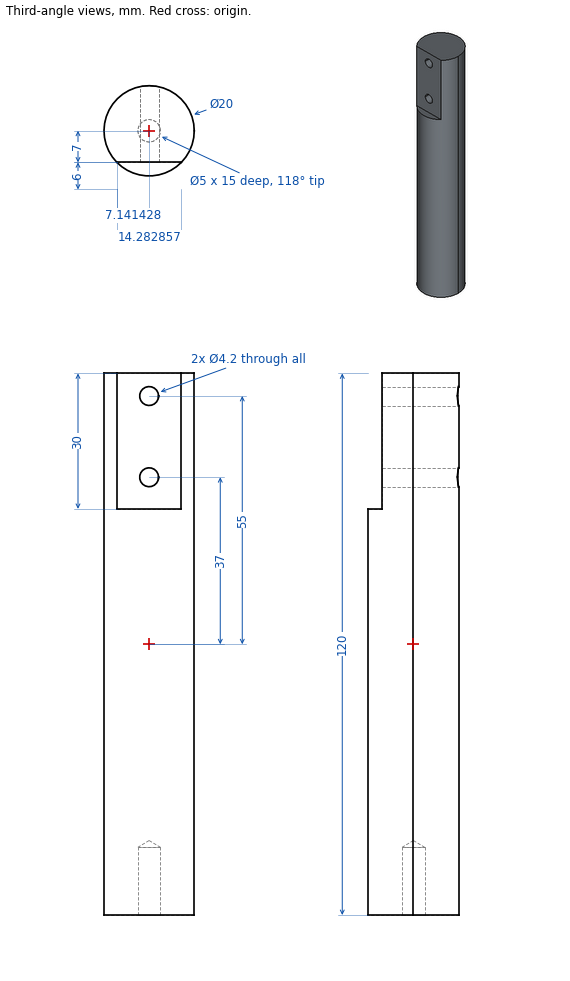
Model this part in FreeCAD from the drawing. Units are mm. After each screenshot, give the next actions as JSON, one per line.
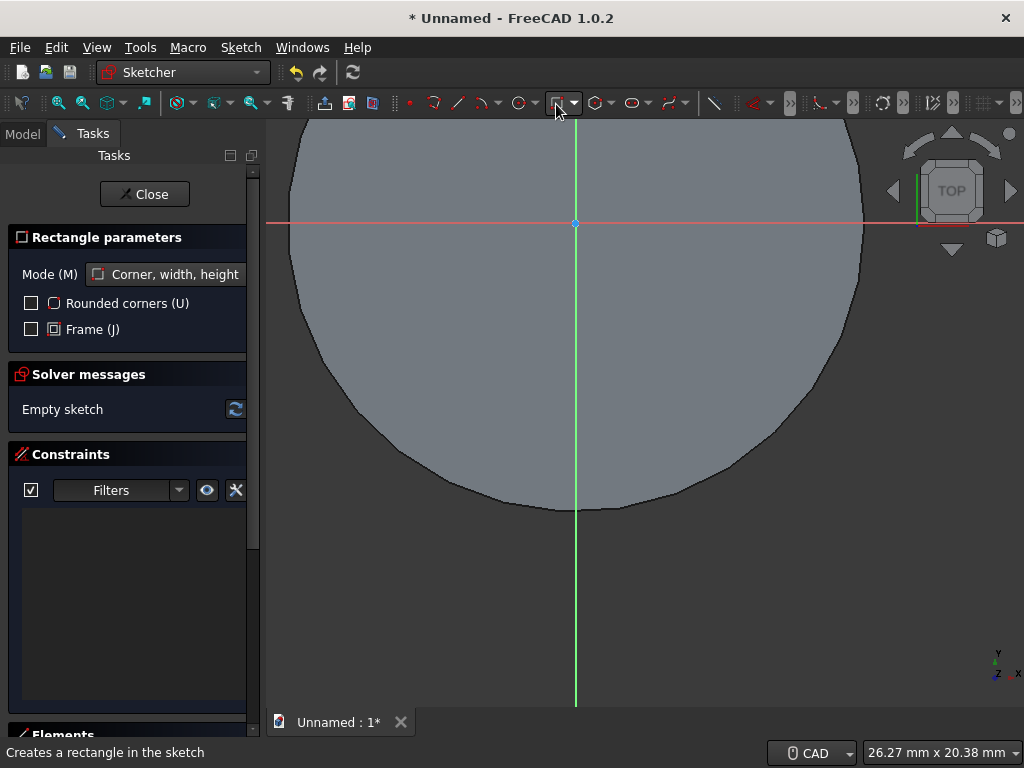
{"action": "left_click", "coordinate": [370, 425]}
{"action": "left_click", "coordinate": [782, 598]}
{"action": "key", "text": "Escape"}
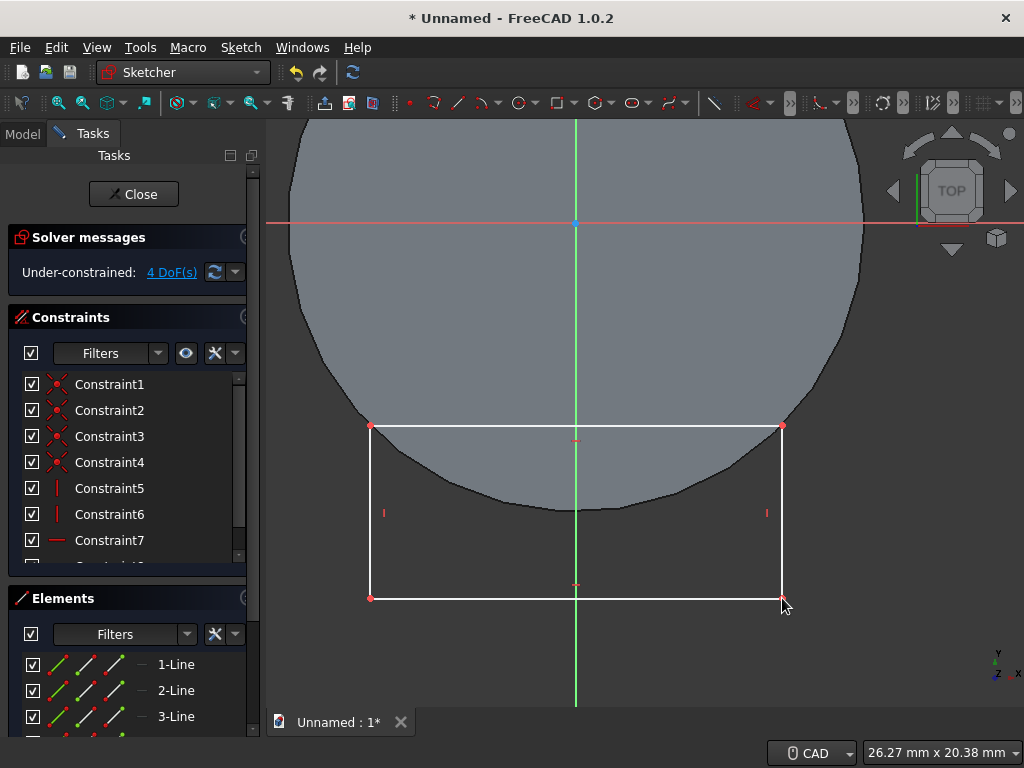
{"action": "left_click", "coordinate": [754, 104]}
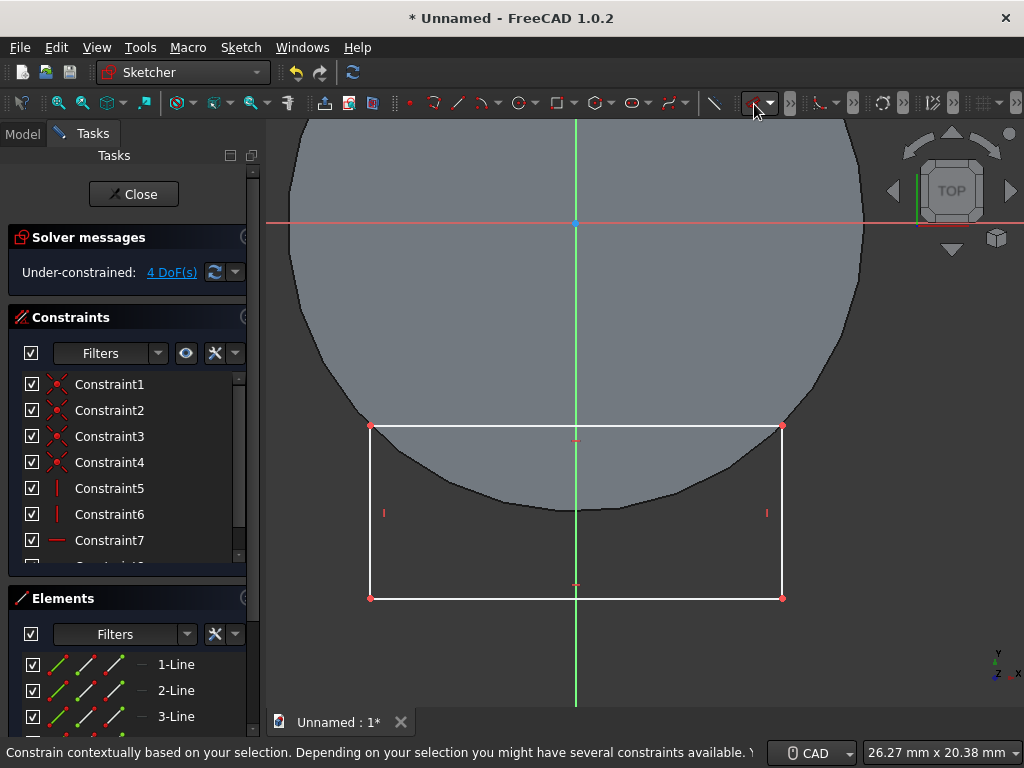
{"action": "left_click", "coordinate": [370, 478]}
{"action": "left_click", "coordinate": [336, 513]}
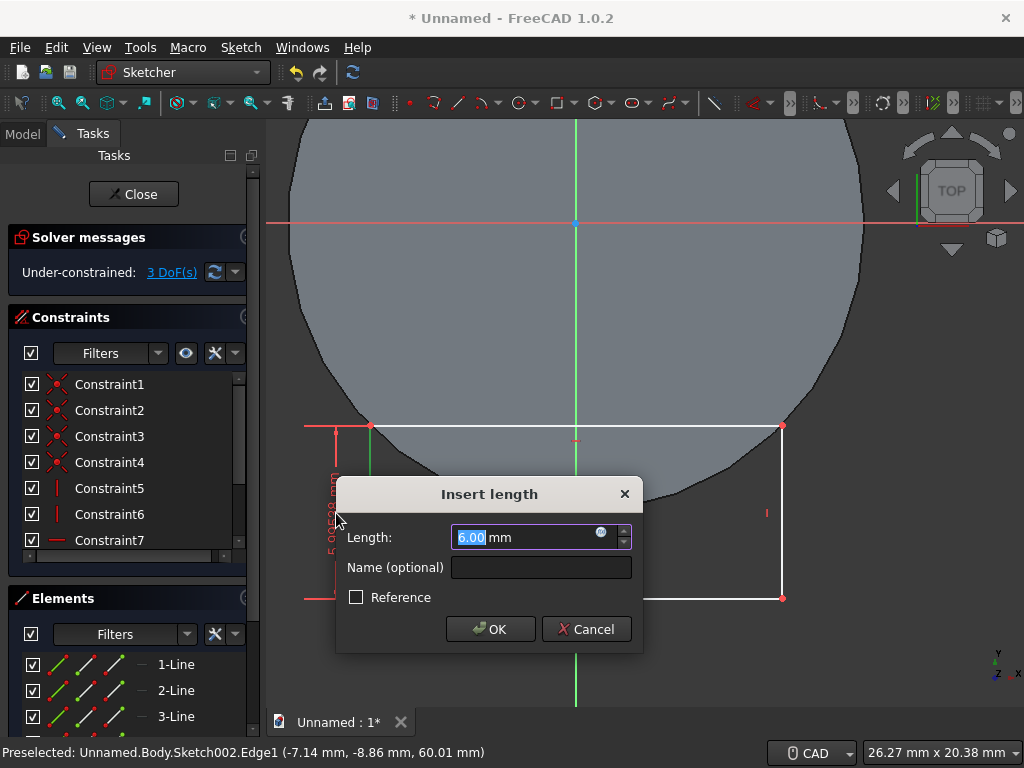
{"action": "type", "text": "6"}
{"action": "key", "text": "Return"}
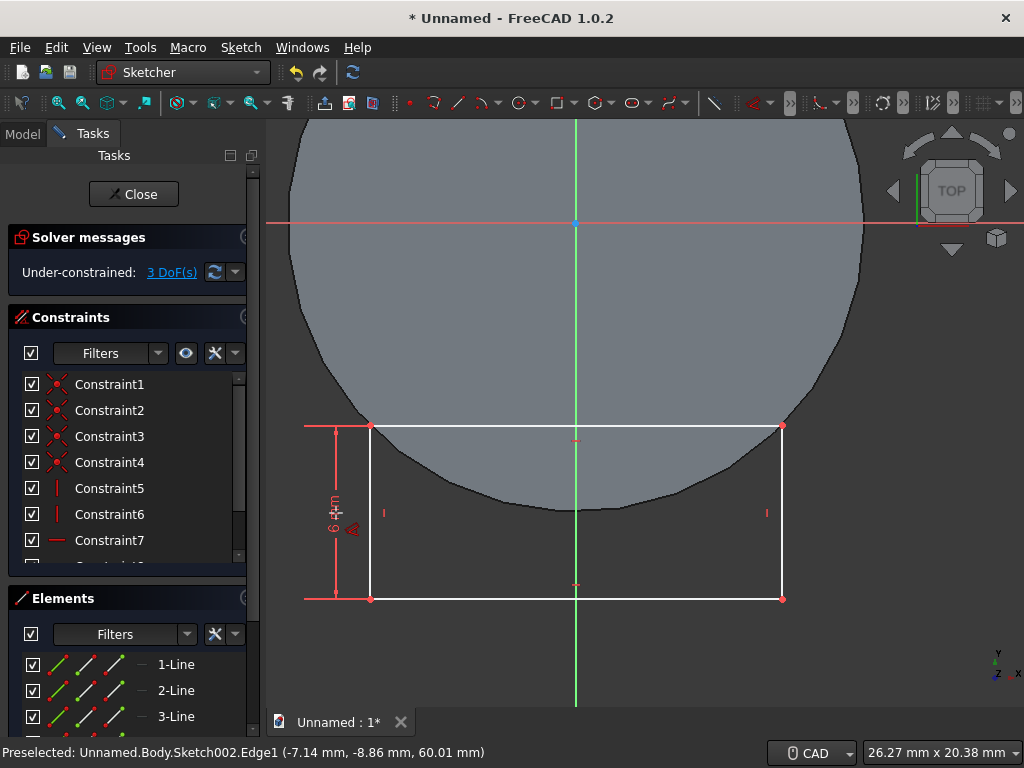
{"action": "left_click", "coordinate": [370, 426]}
{"action": "left_click", "coordinate": [336, 325]}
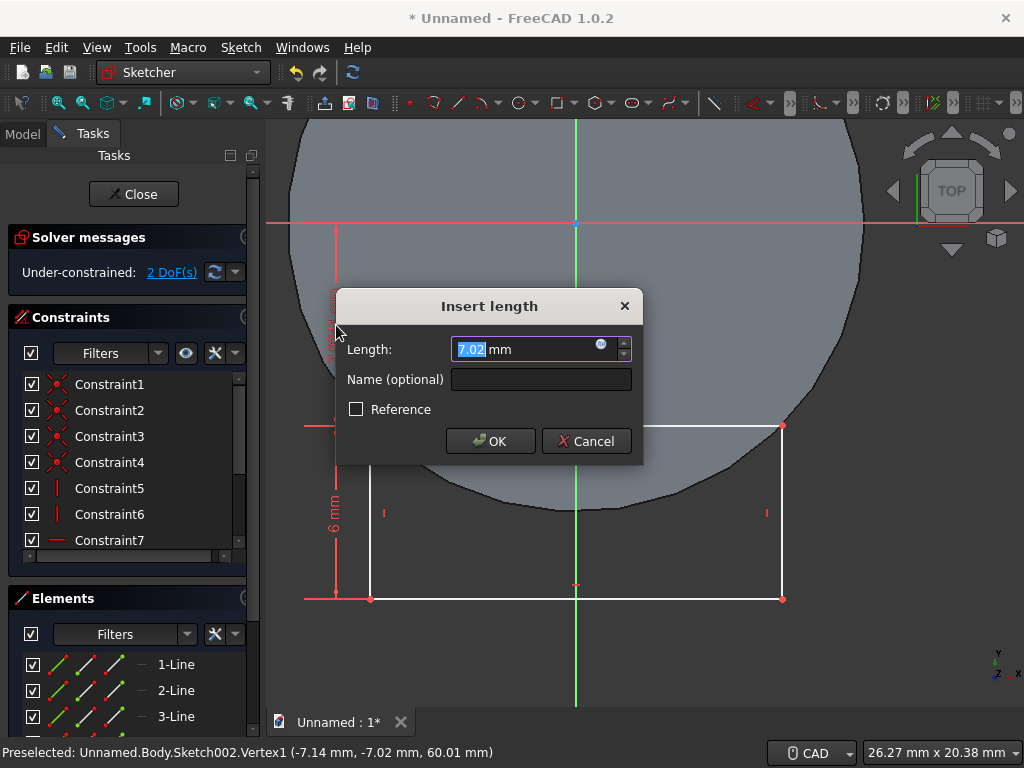
{"action": "type", "text": "7"}
{"action": "key", "text": "Return"}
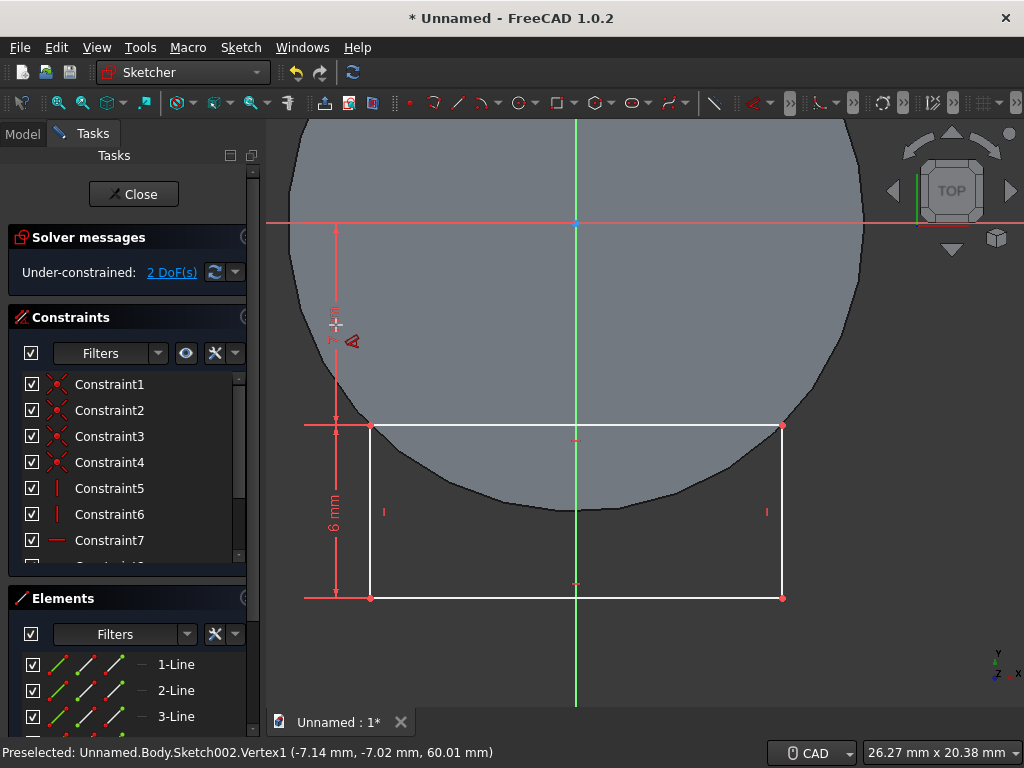
{"action": "left_click", "coordinate": [494, 598]}
{"action": "left_click", "coordinate": [481, 632]}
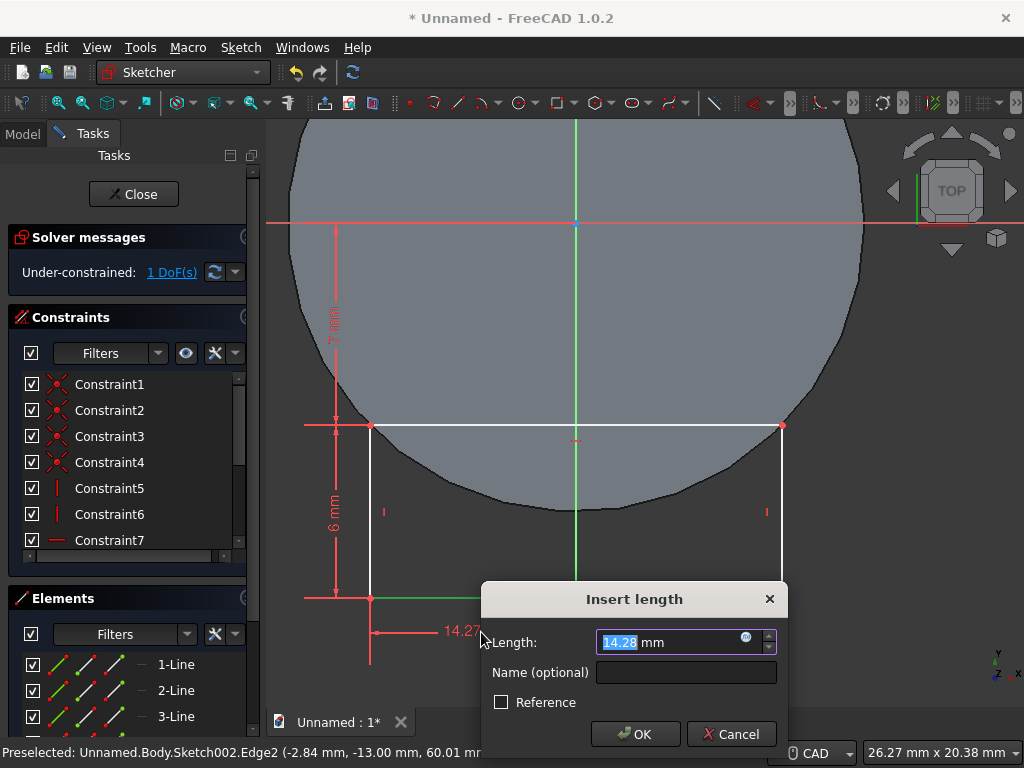
{"action": "type", "text": "14.282857"}
{"action": "key", "text": "Return"}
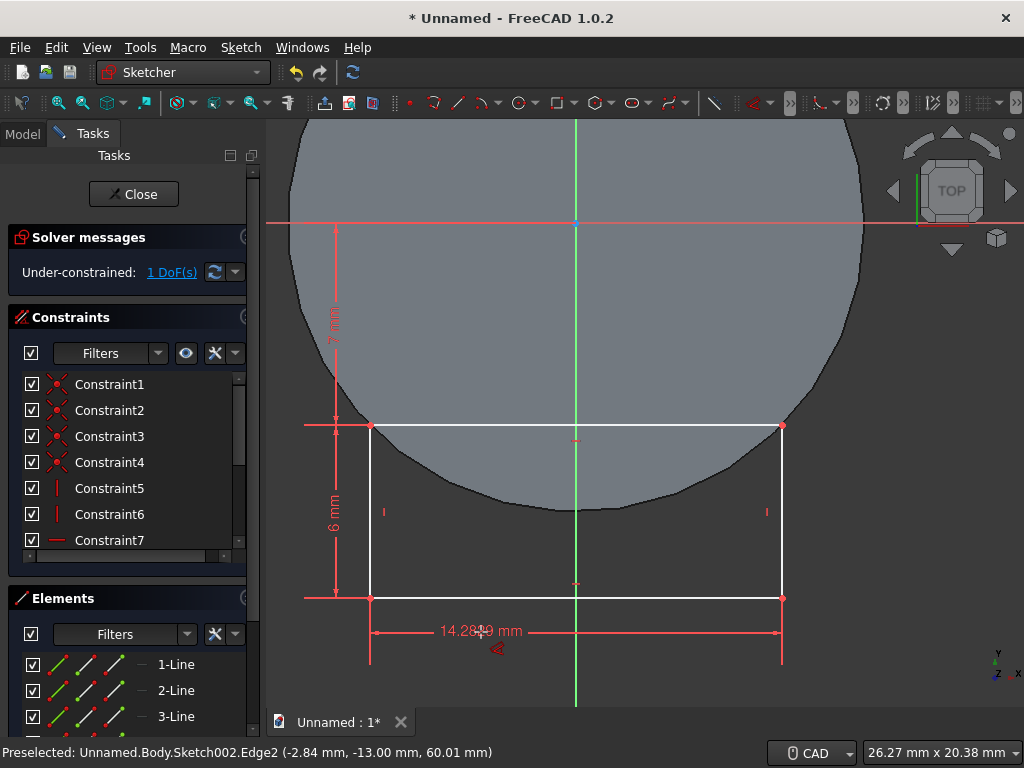
{"action": "left_click", "coordinate": [370, 425]}
{"action": "left_click", "coordinate": [473, 189]}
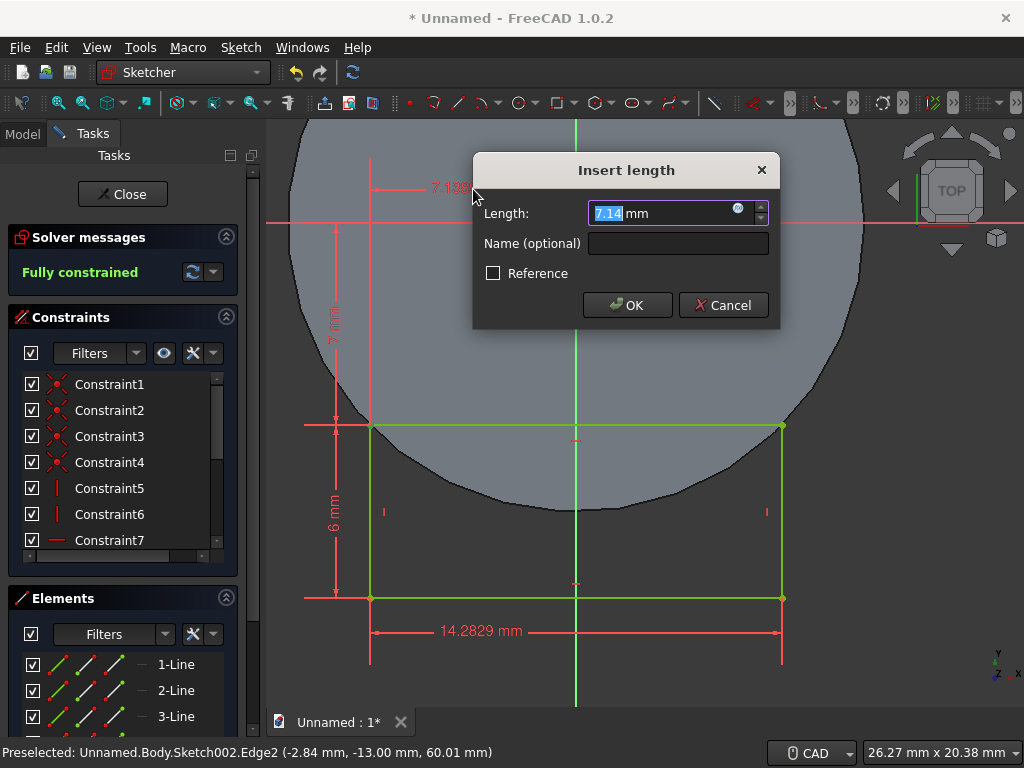
{"action": "type", "text": "7.141428"}
{"action": "key", "text": "Return"}
{"action": "key", "text": "Escape"}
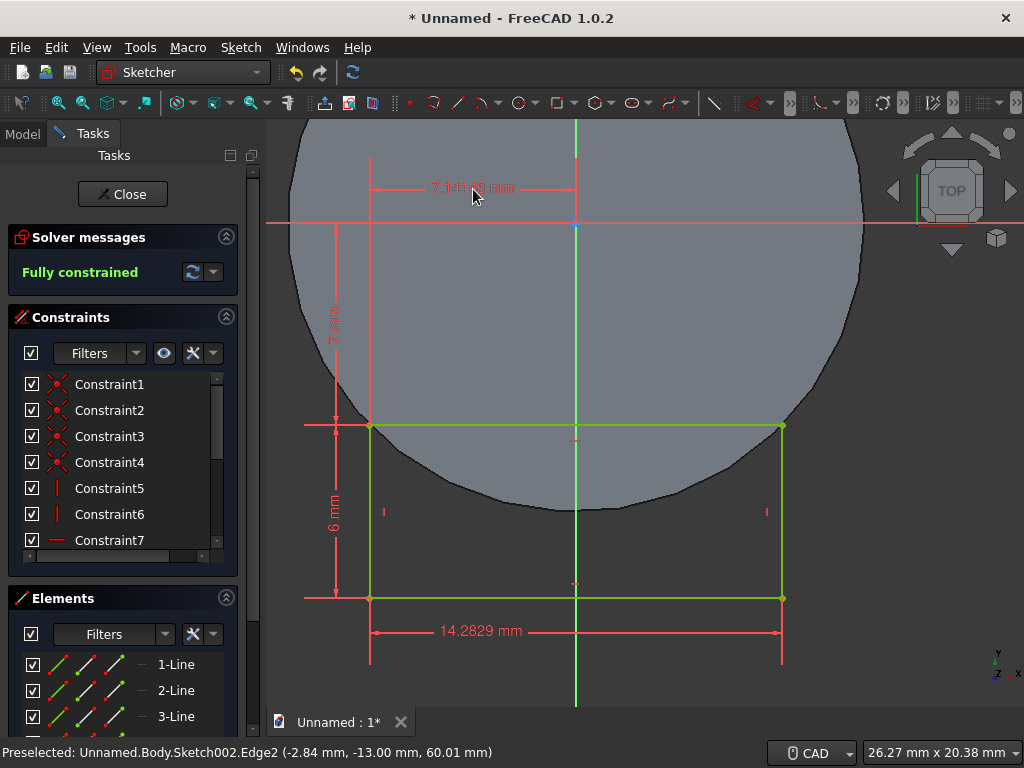
{"action": "left_click", "coordinate": [123, 194]}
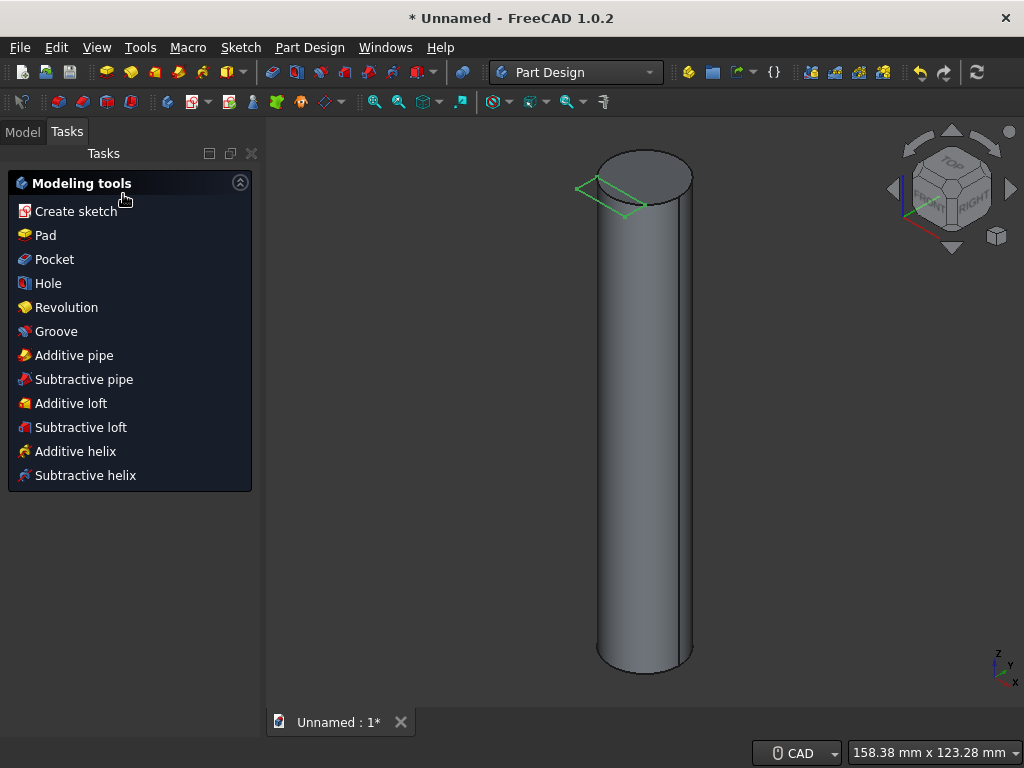
{"action": "left_click", "coordinate": [274, 72]}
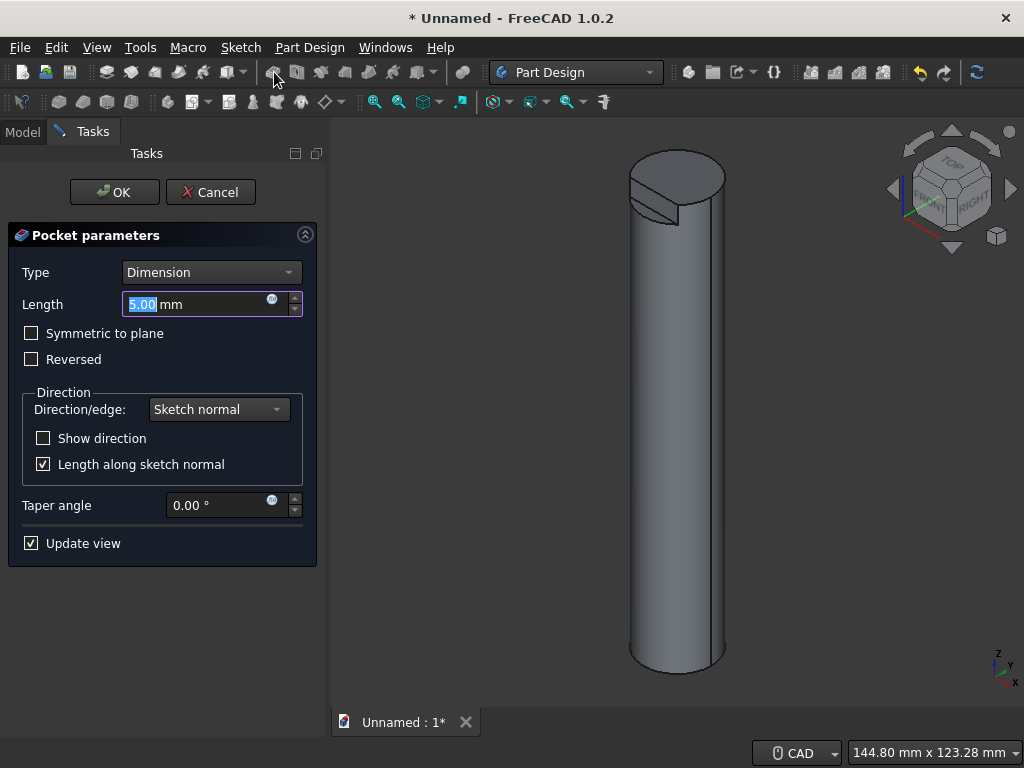
{"action": "type", "text": "30"}
{"action": "key", "text": "Tab"}